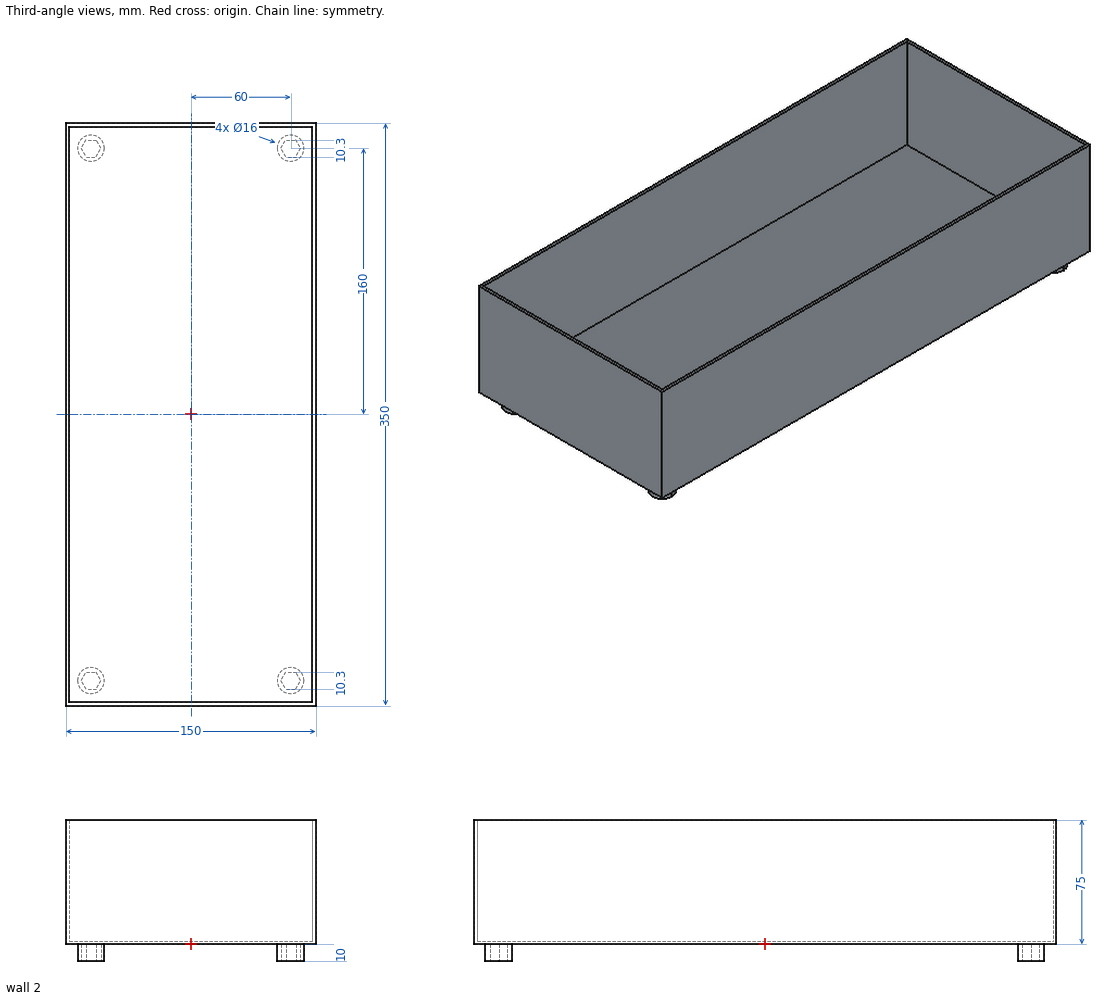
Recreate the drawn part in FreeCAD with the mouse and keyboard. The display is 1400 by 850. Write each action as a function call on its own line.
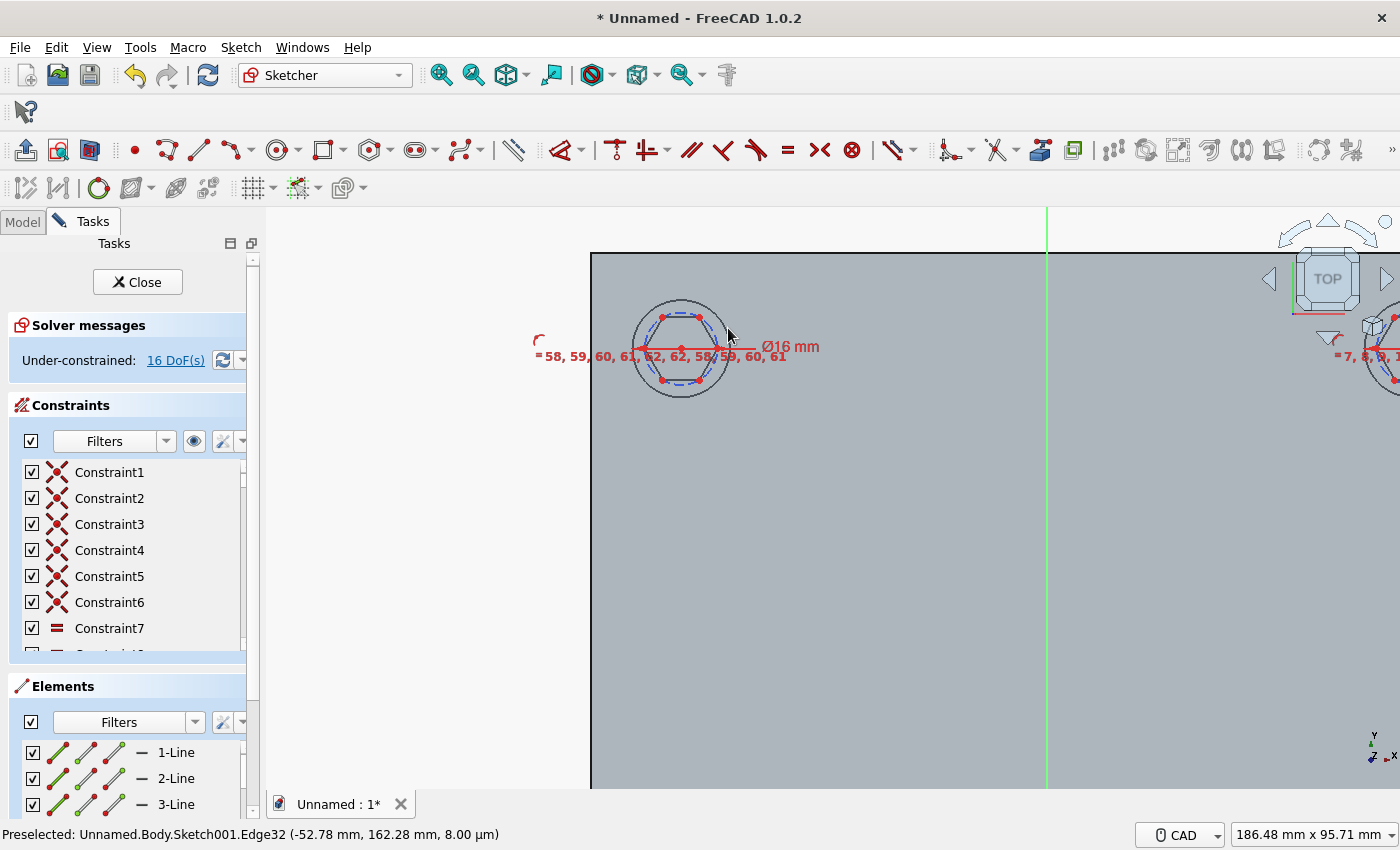
scroll(708, 336, down, 9)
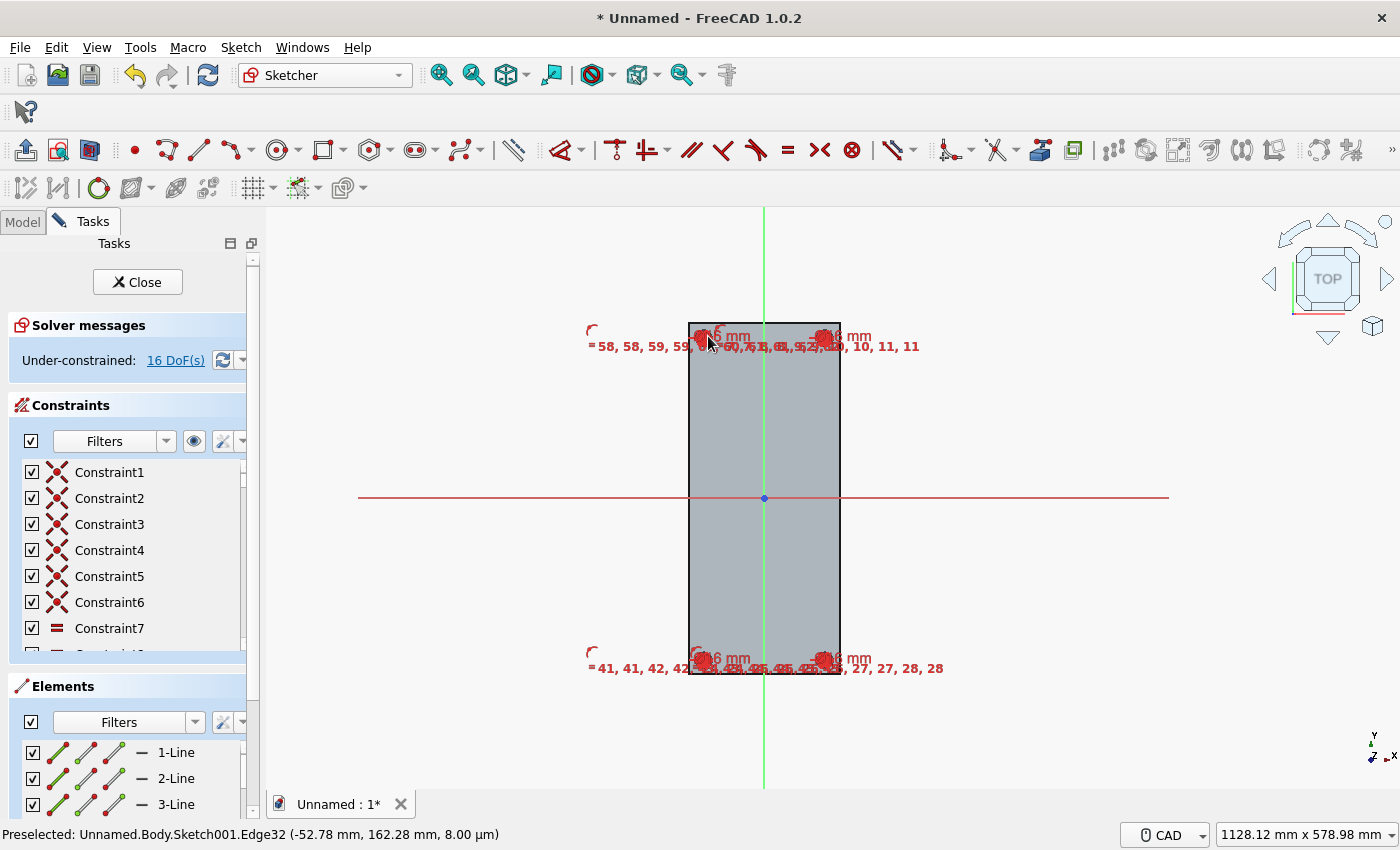
scroll(825, 333, up, 14)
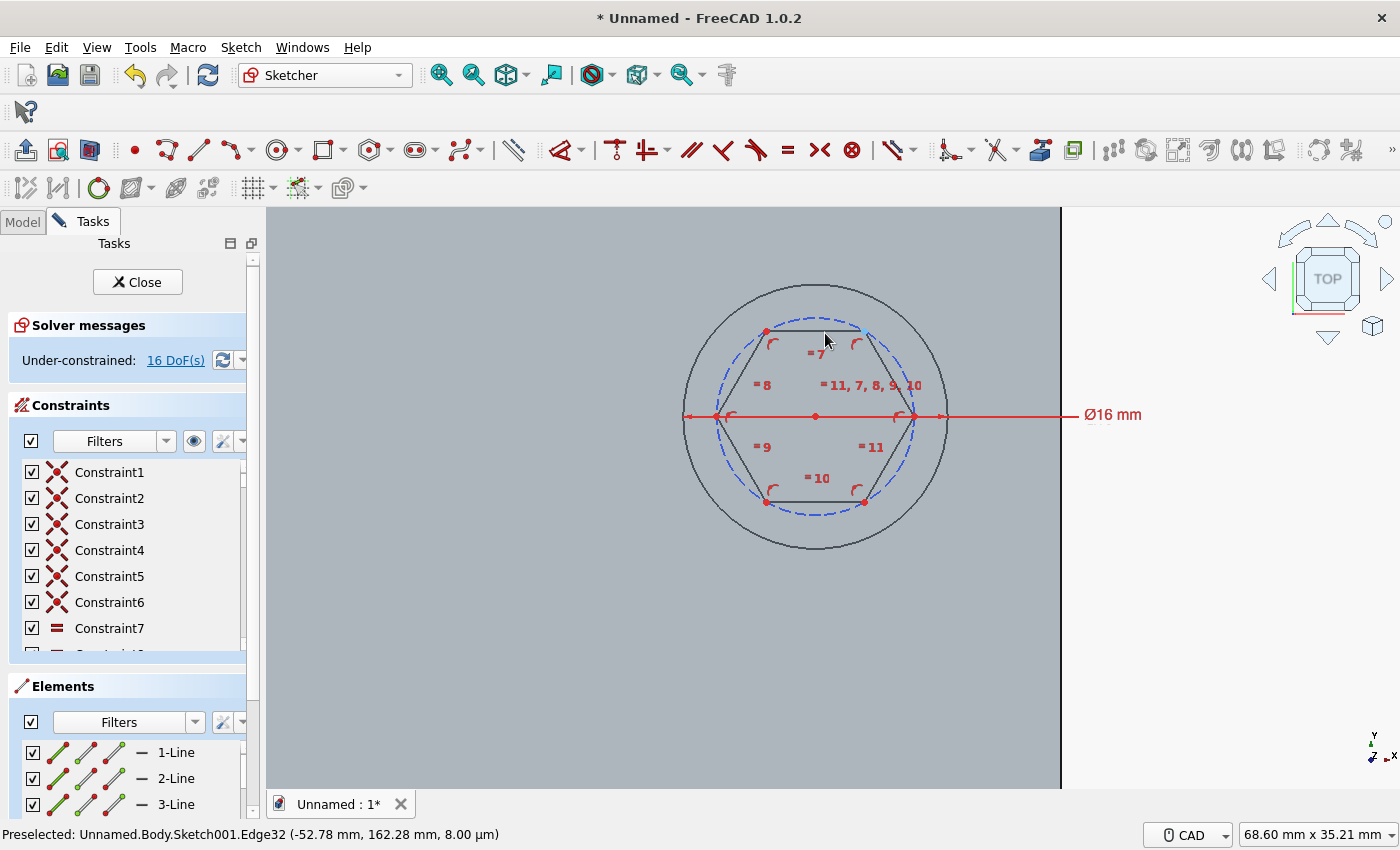
click(815, 331)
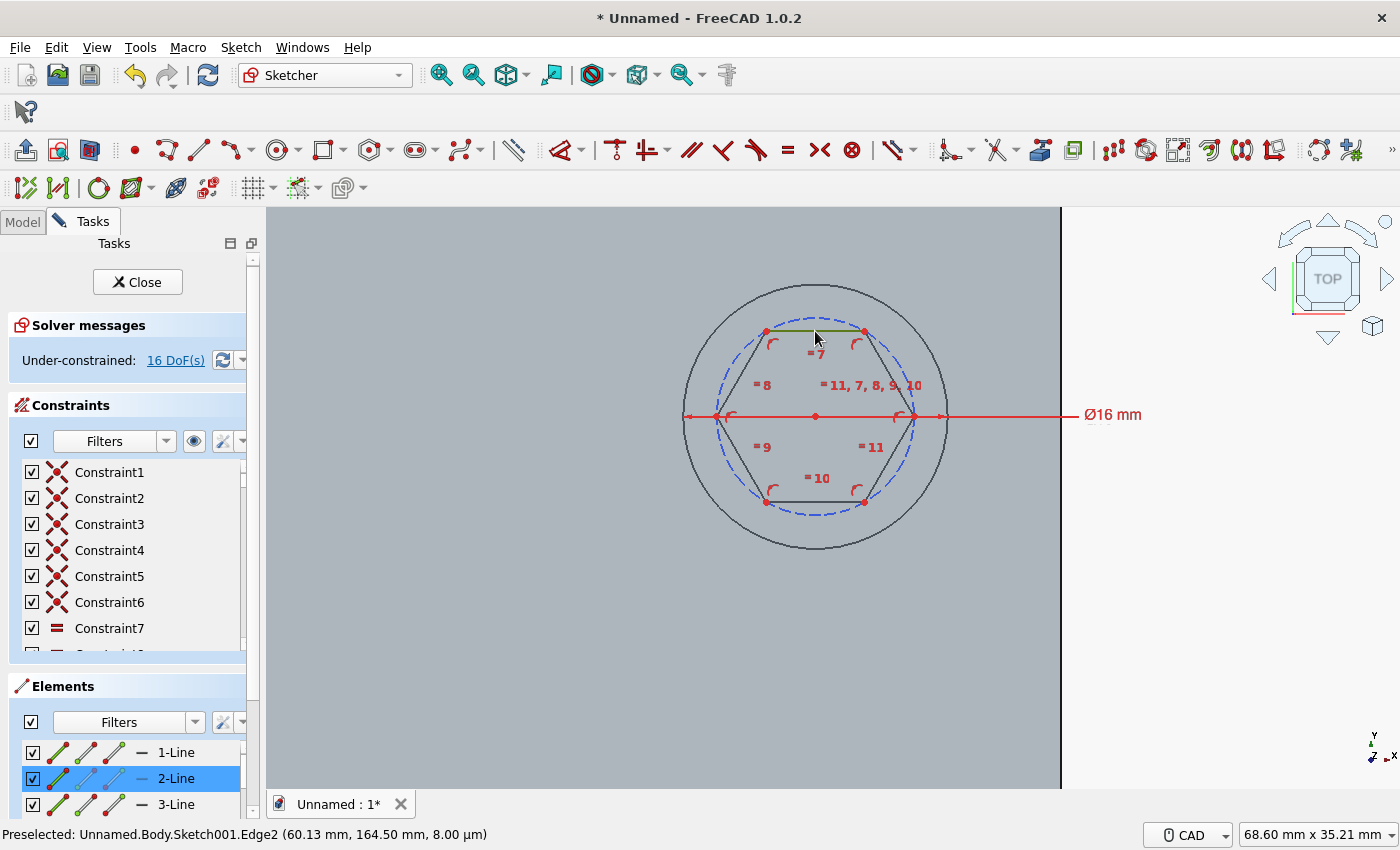
key(h)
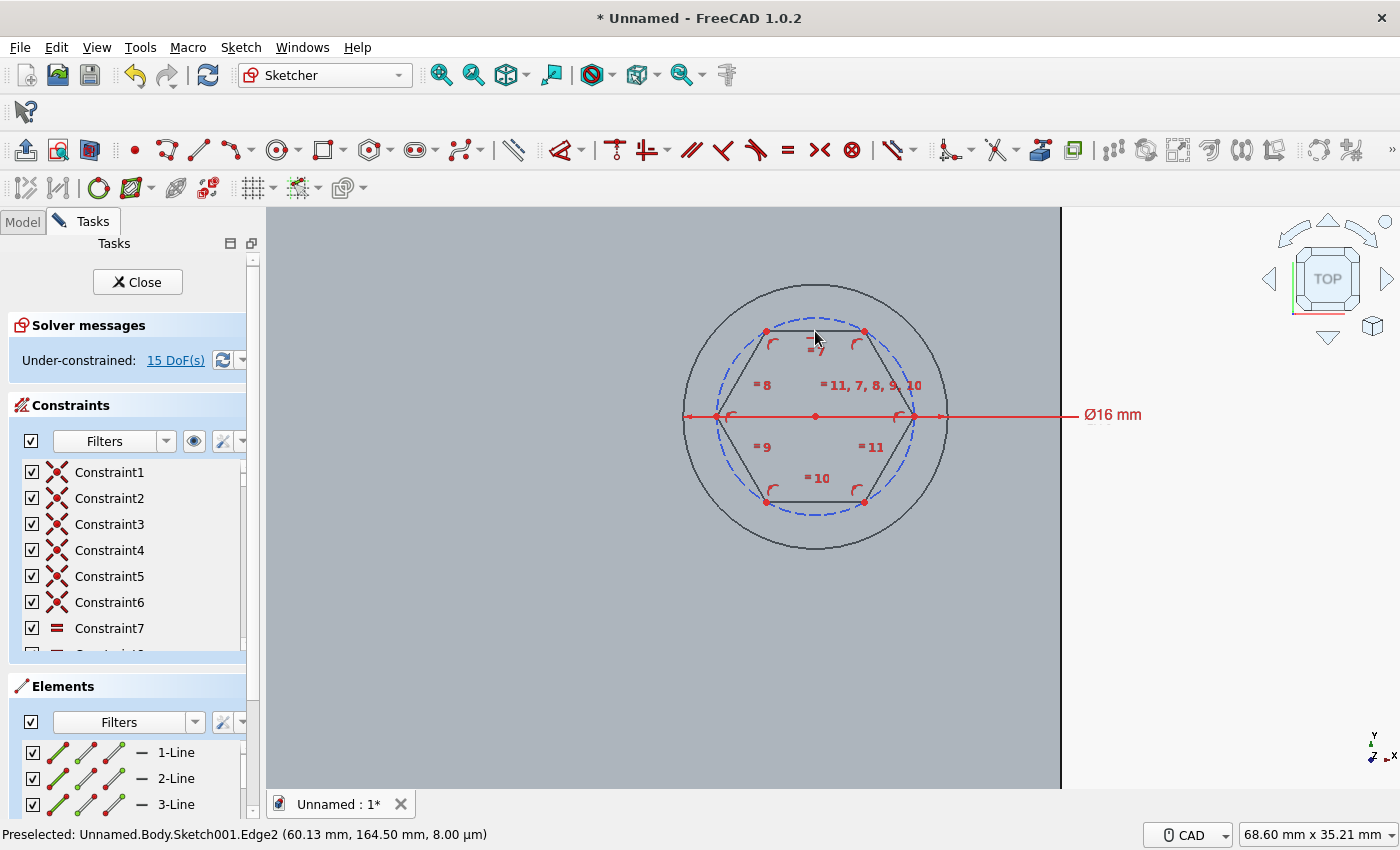
scroll(826, 333, down, 14)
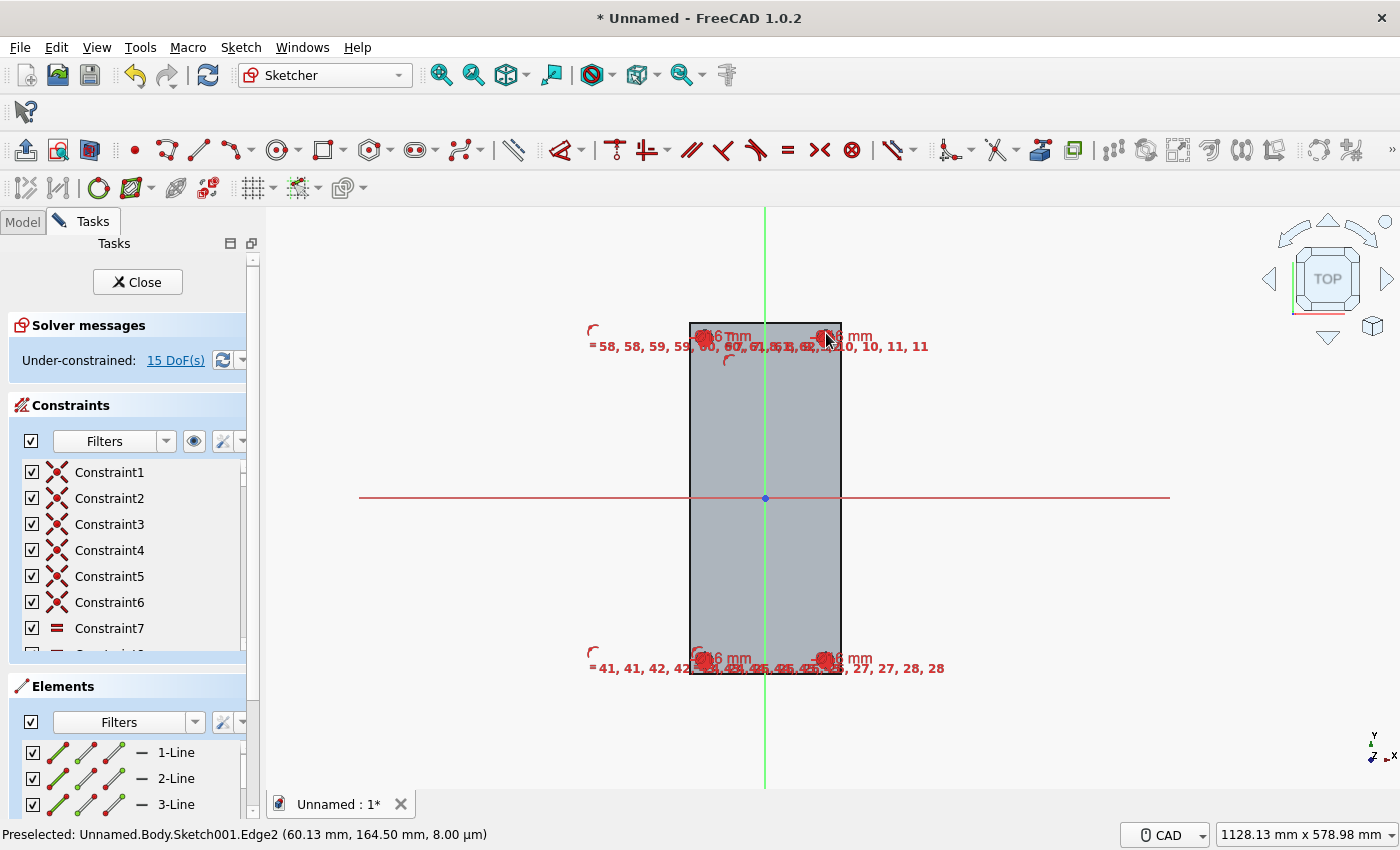
scroll(827, 655, up, 14)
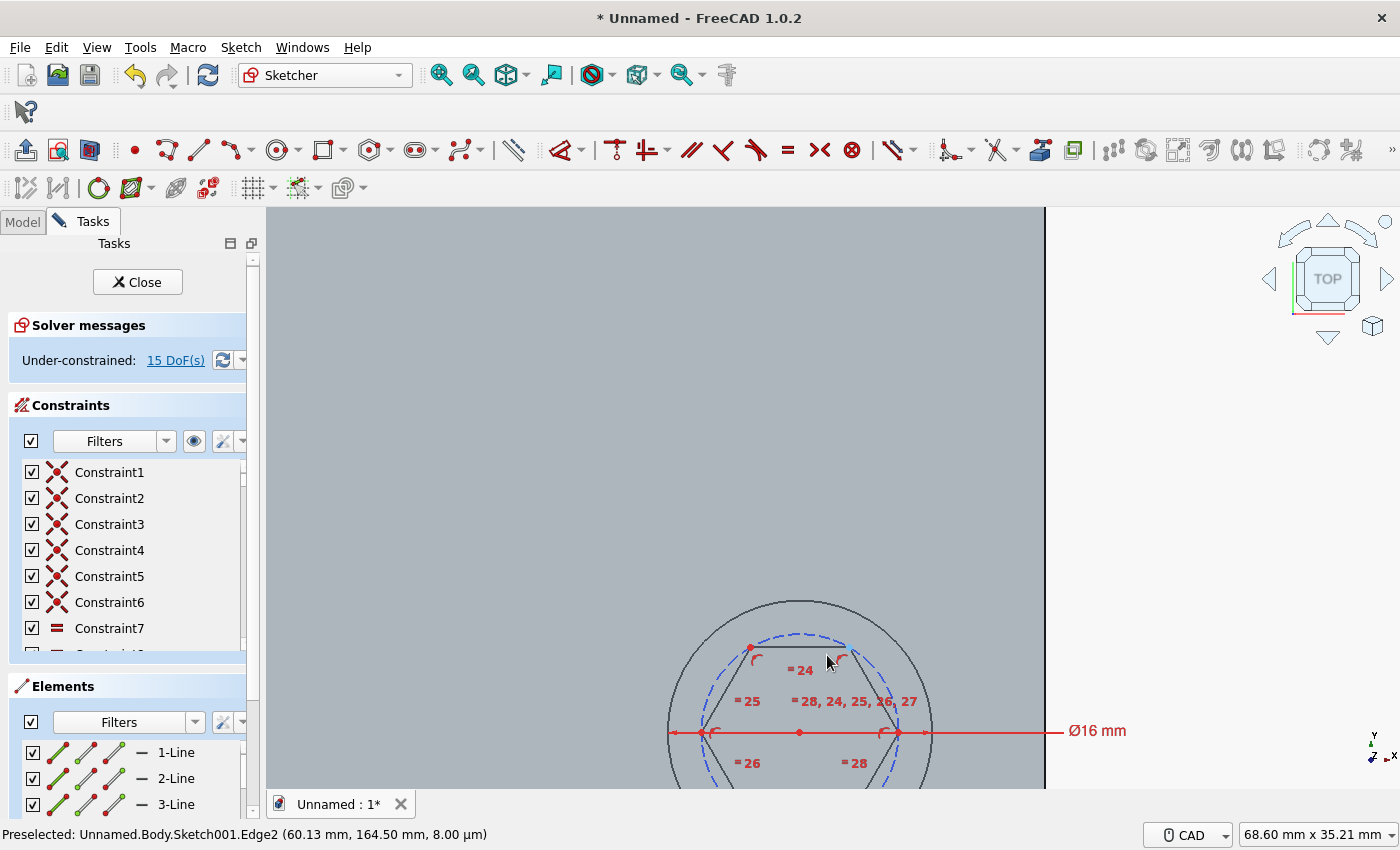
click(820, 647)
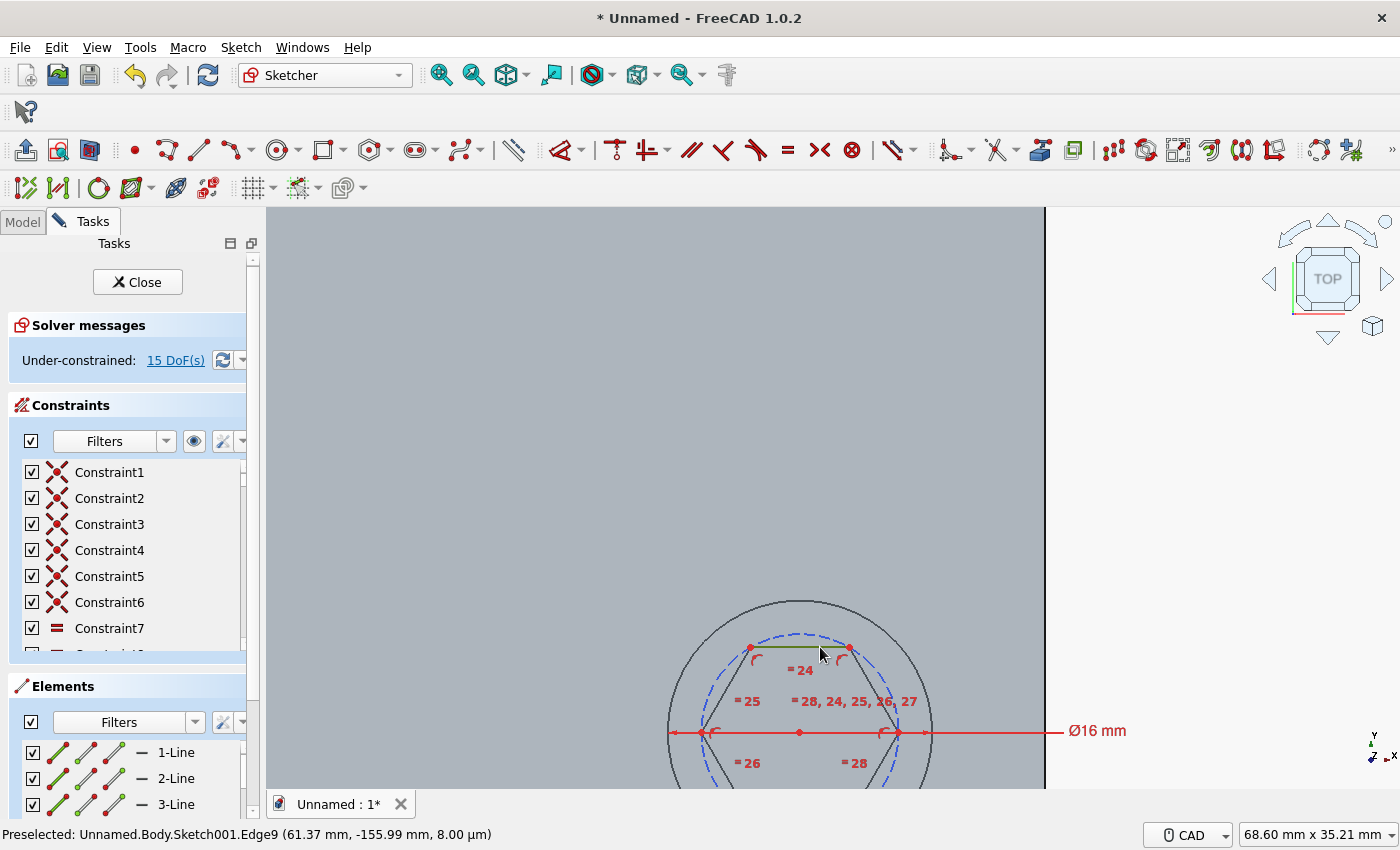
click(670, 150)